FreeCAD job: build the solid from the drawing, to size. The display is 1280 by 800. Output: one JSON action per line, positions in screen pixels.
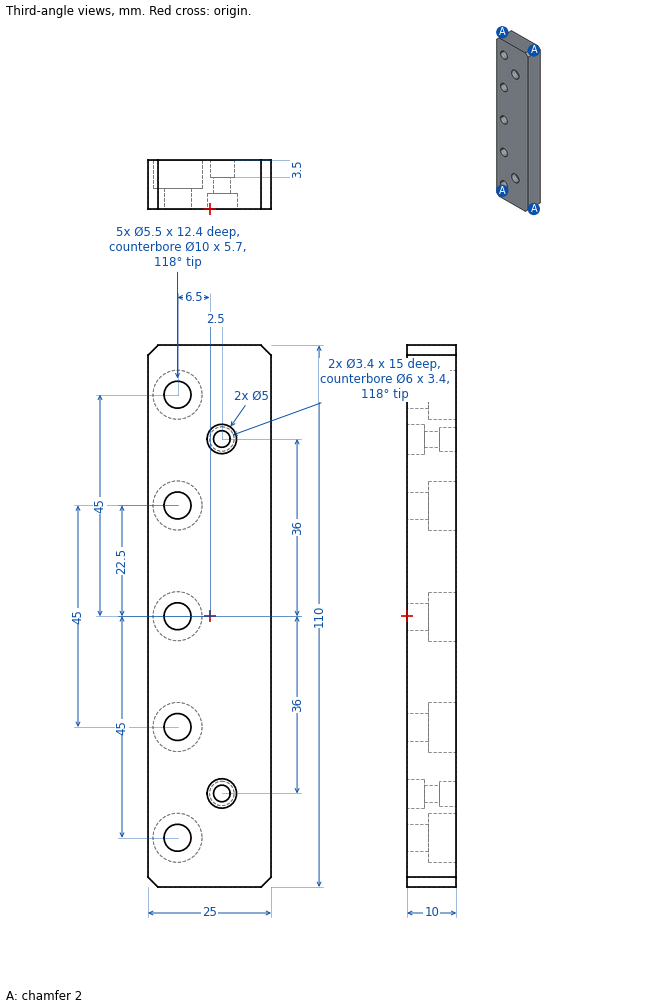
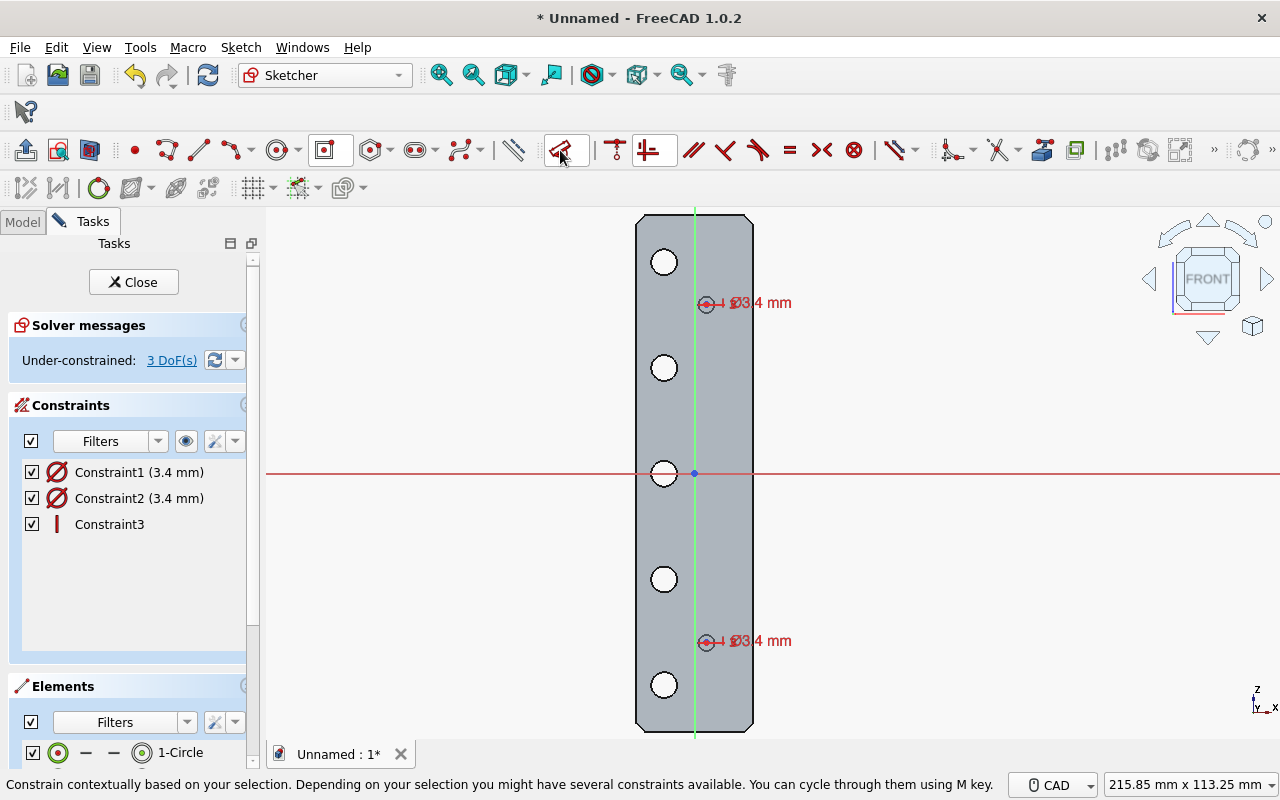
{"action": "left_click", "coordinate": [706, 305]}
{"action": "left_click", "coordinate": [661, 389]}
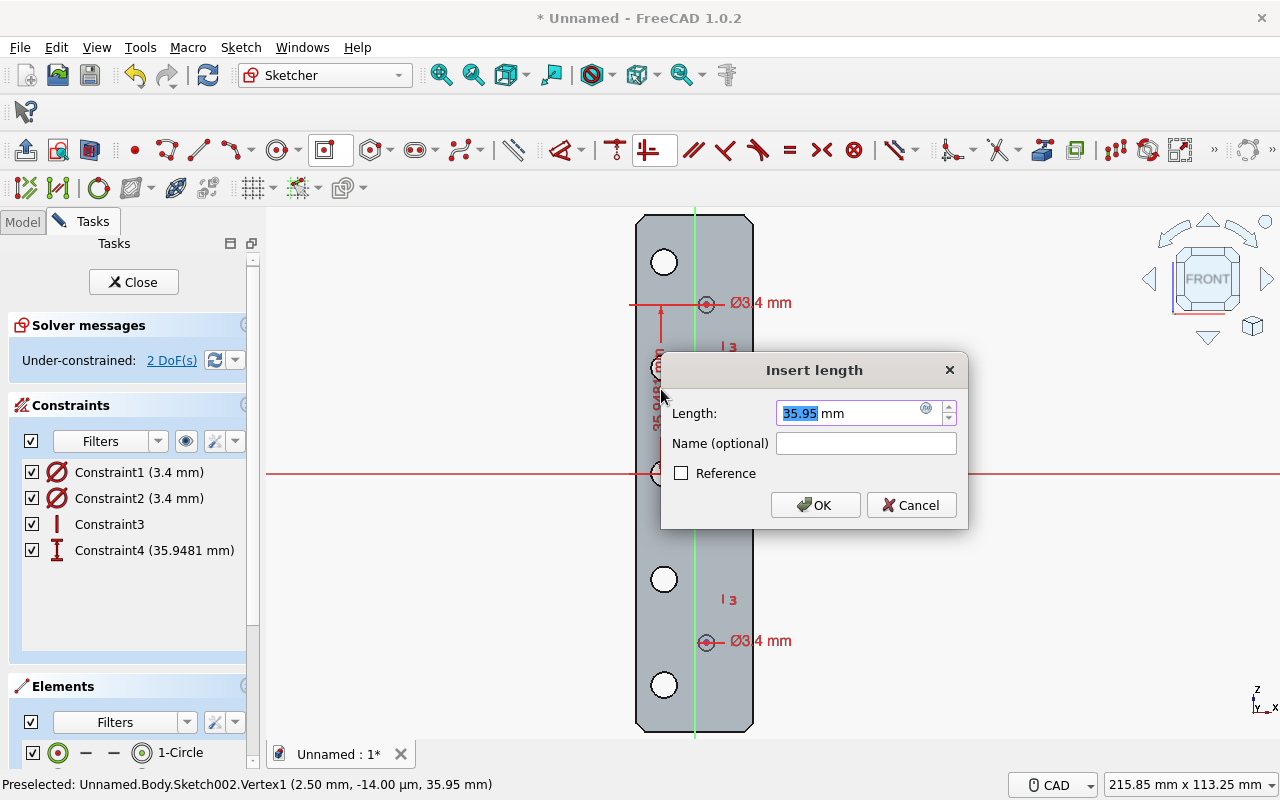
{"action": "type", "text": "36"}
{"action": "key", "text": "Return"}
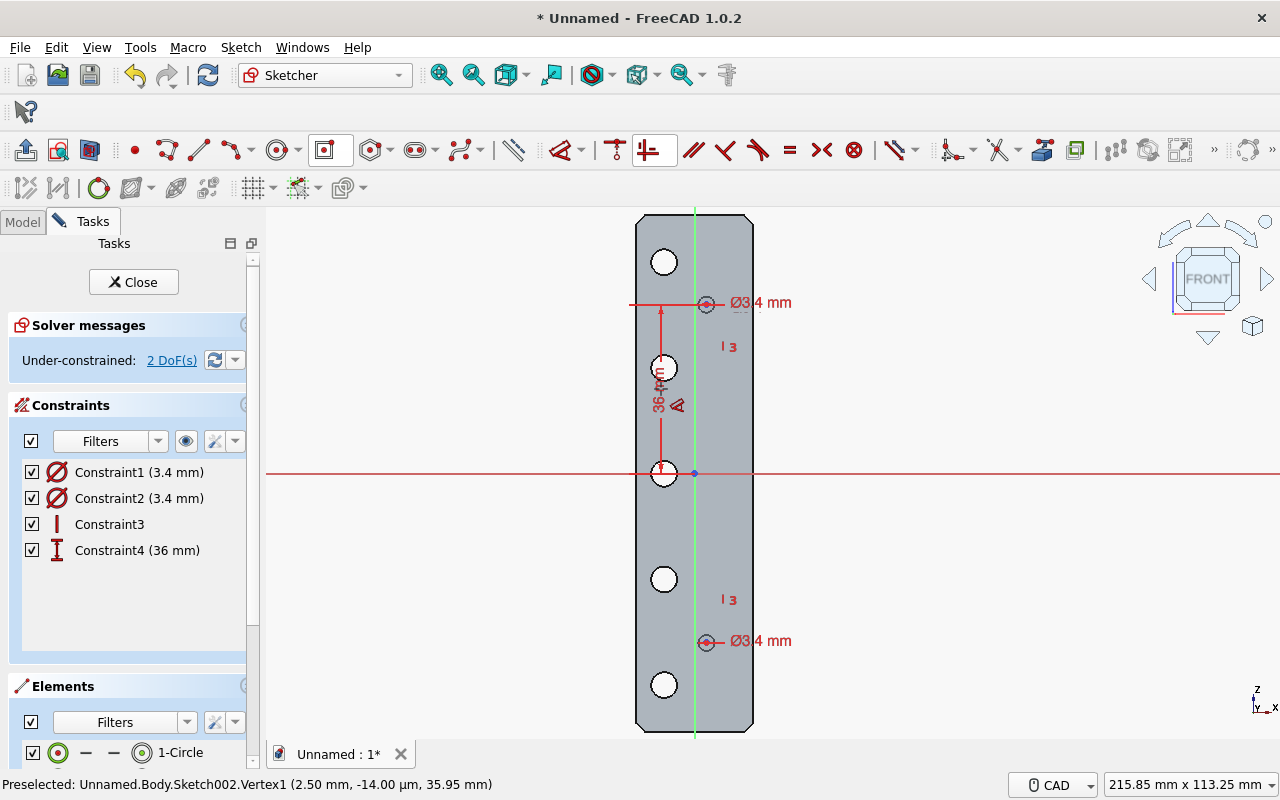
{"action": "left_click", "coordinate": [706, 643]}
{"action": "left_click", "coordinate": [661, 558]}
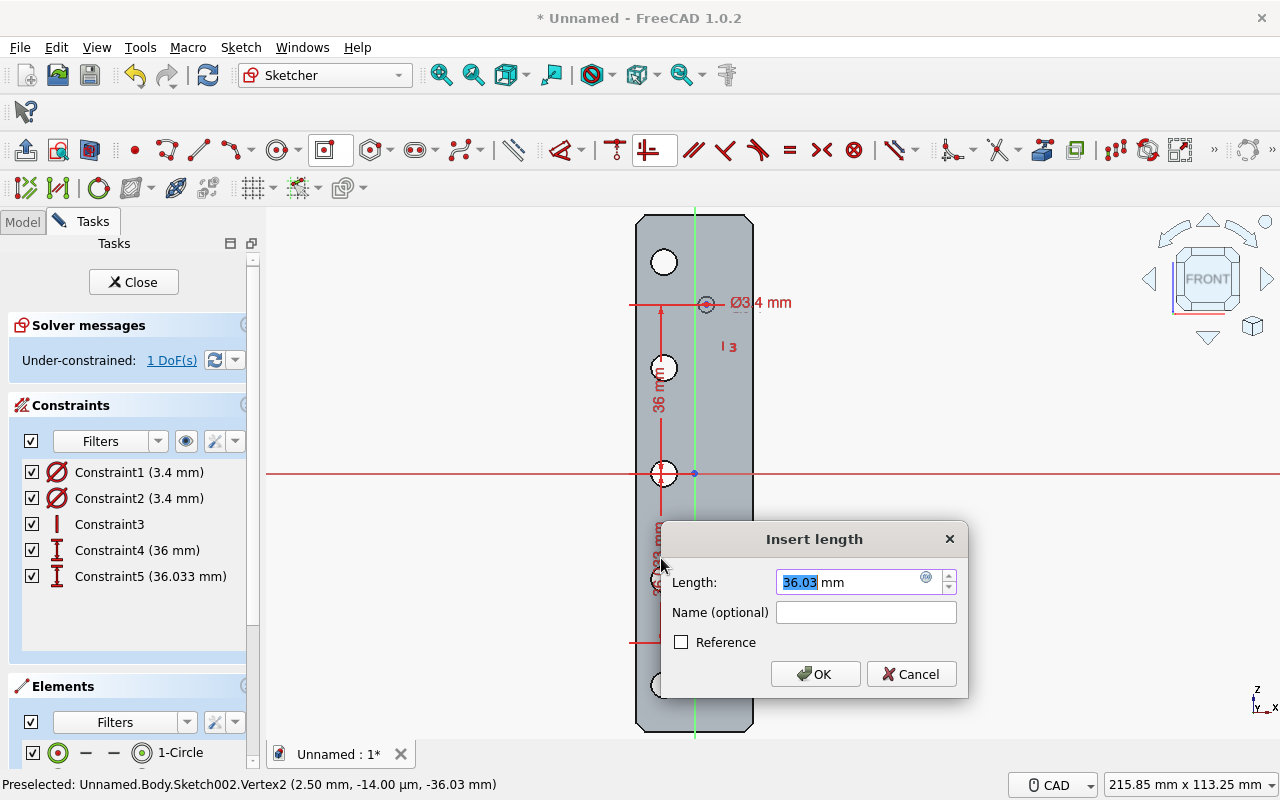
{"action": "type", "text": "36"}
{"action": "key", "text": "Return"}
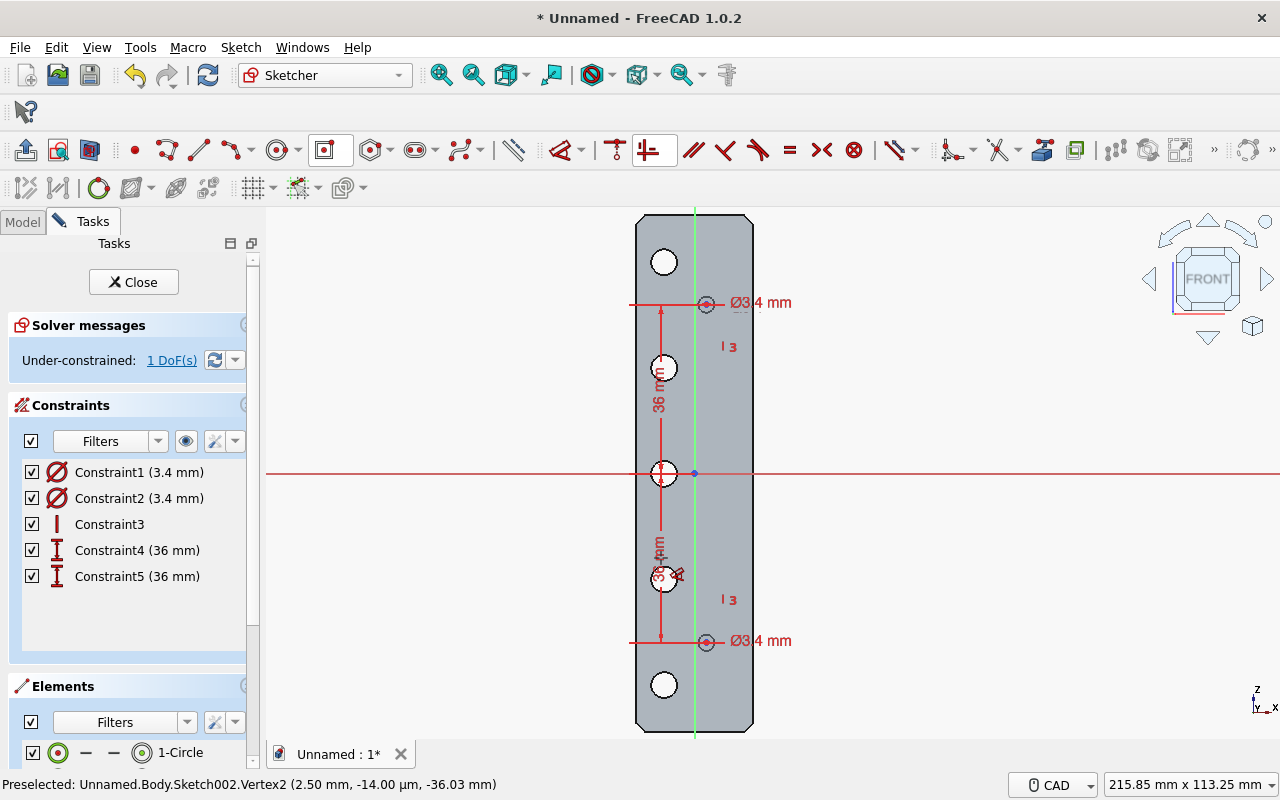
{"action": "scroll", "coordinate": [706, 305], "scroll_direction": "up", "scroll_amount": 7}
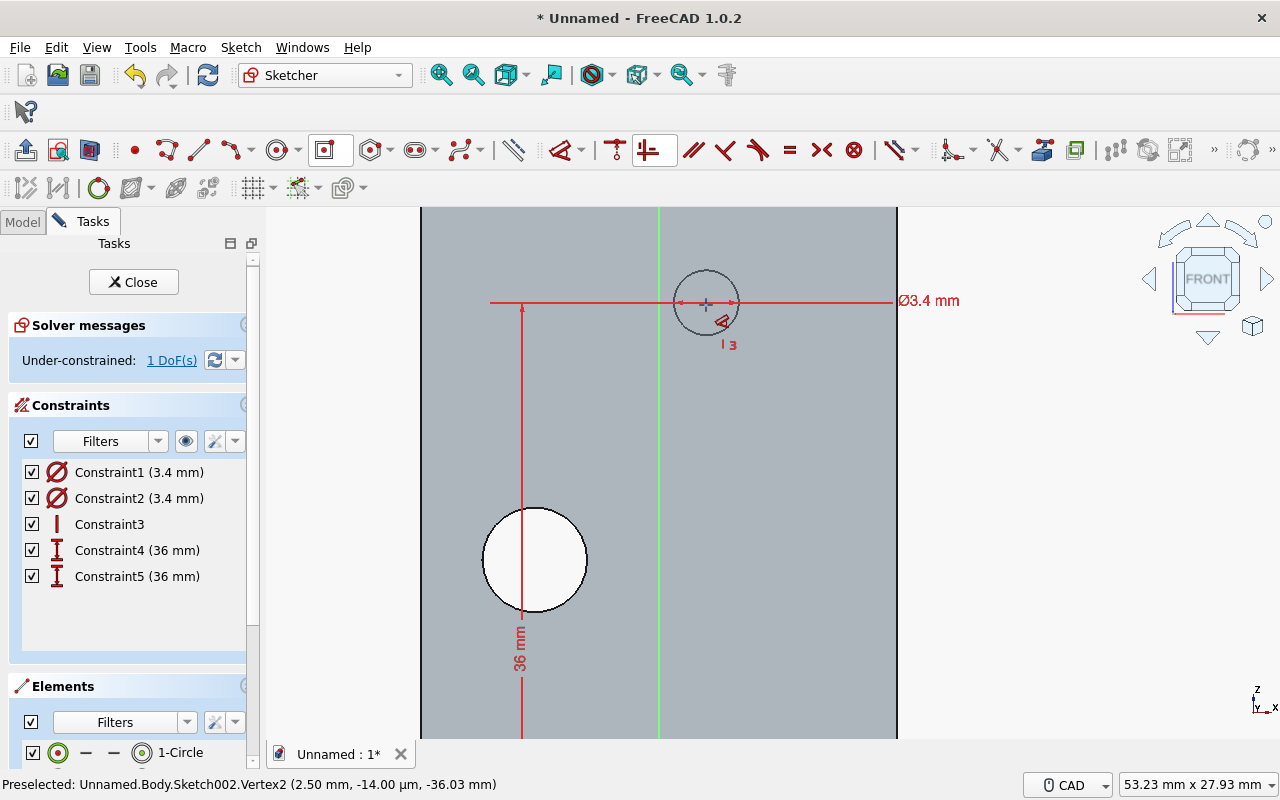
{"action": "left_click", "coordinate": [706, 303]}
{"action": "left_click", "coordinate": [683, 245]}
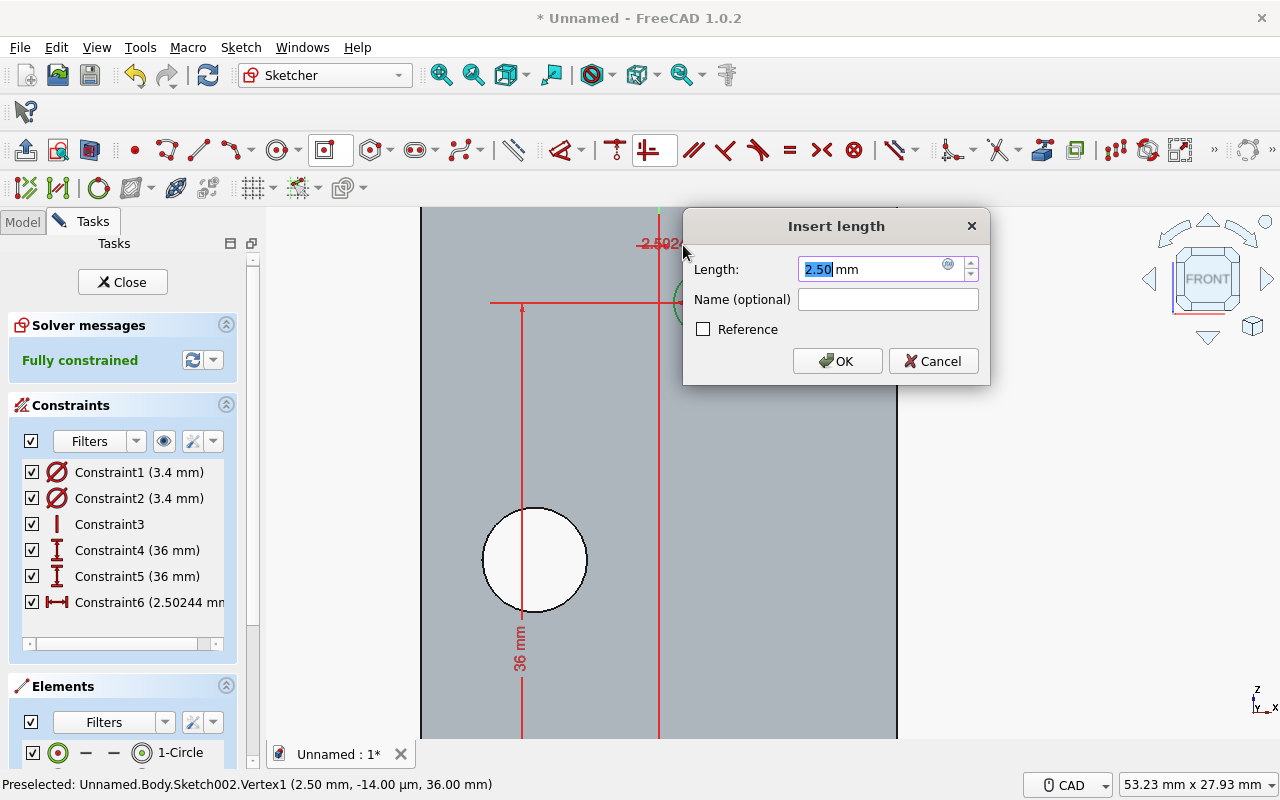
{"action": "type", "text": "2.5"}
{"action": "key", "text": "Return"}
{"action": "key", "text": "Escape"}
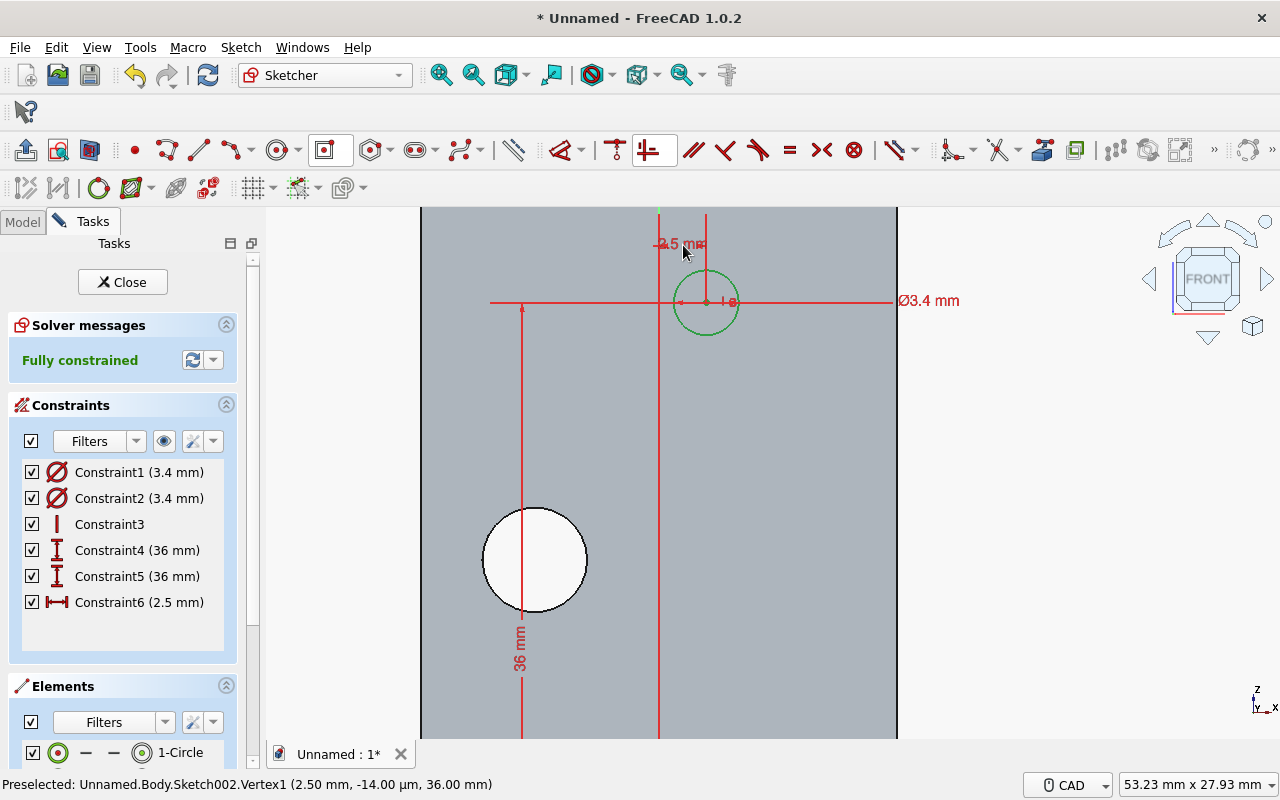
{"action": "left_click", "coordinate": [123, 282]}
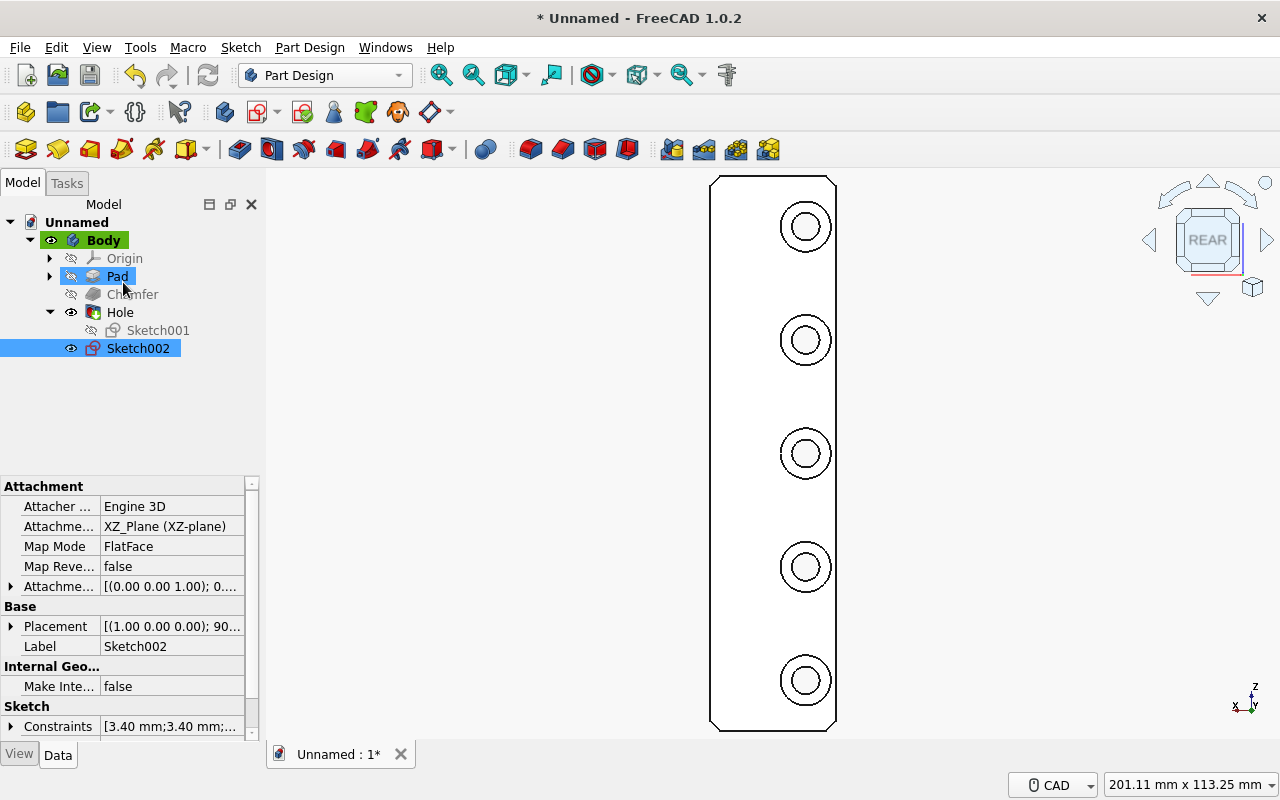
{"action": "left_click", "coordinate": [272, 150]}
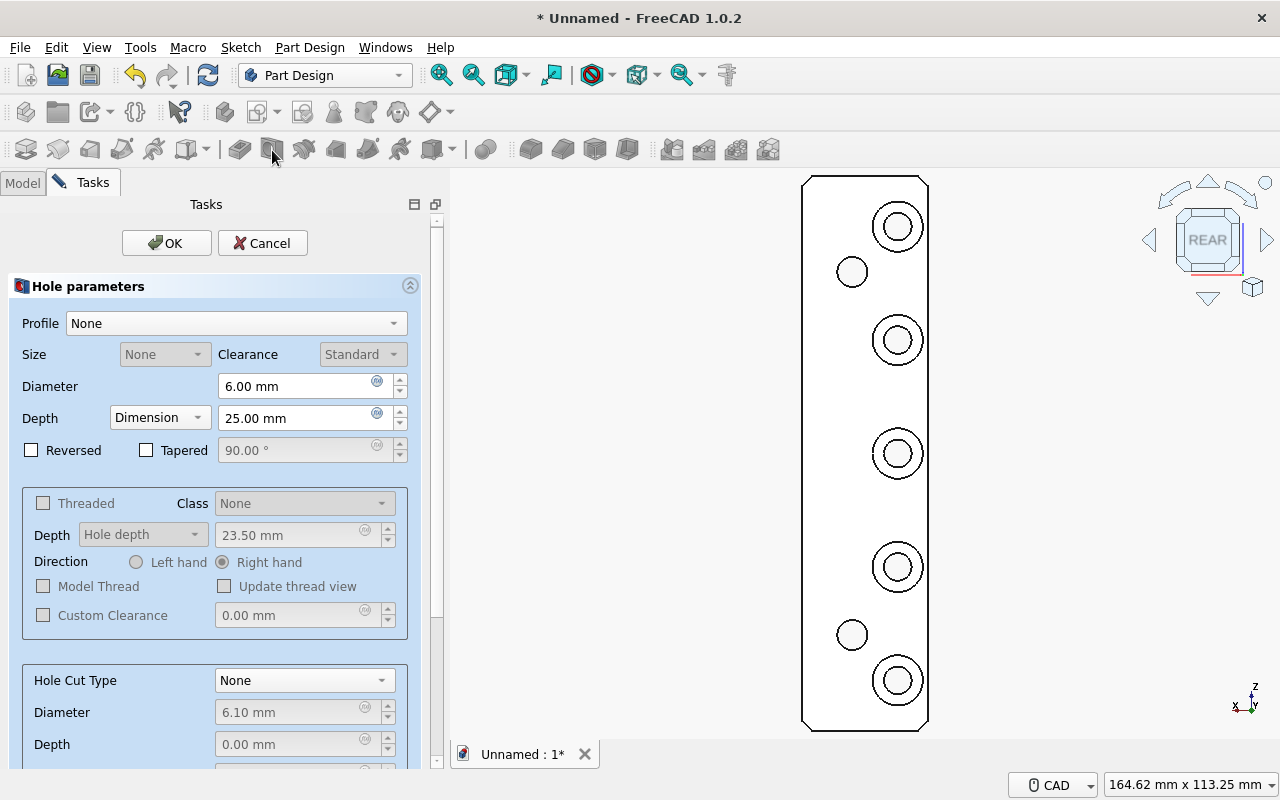
{"action": "triple_click", "coordinate": [305, 386]}